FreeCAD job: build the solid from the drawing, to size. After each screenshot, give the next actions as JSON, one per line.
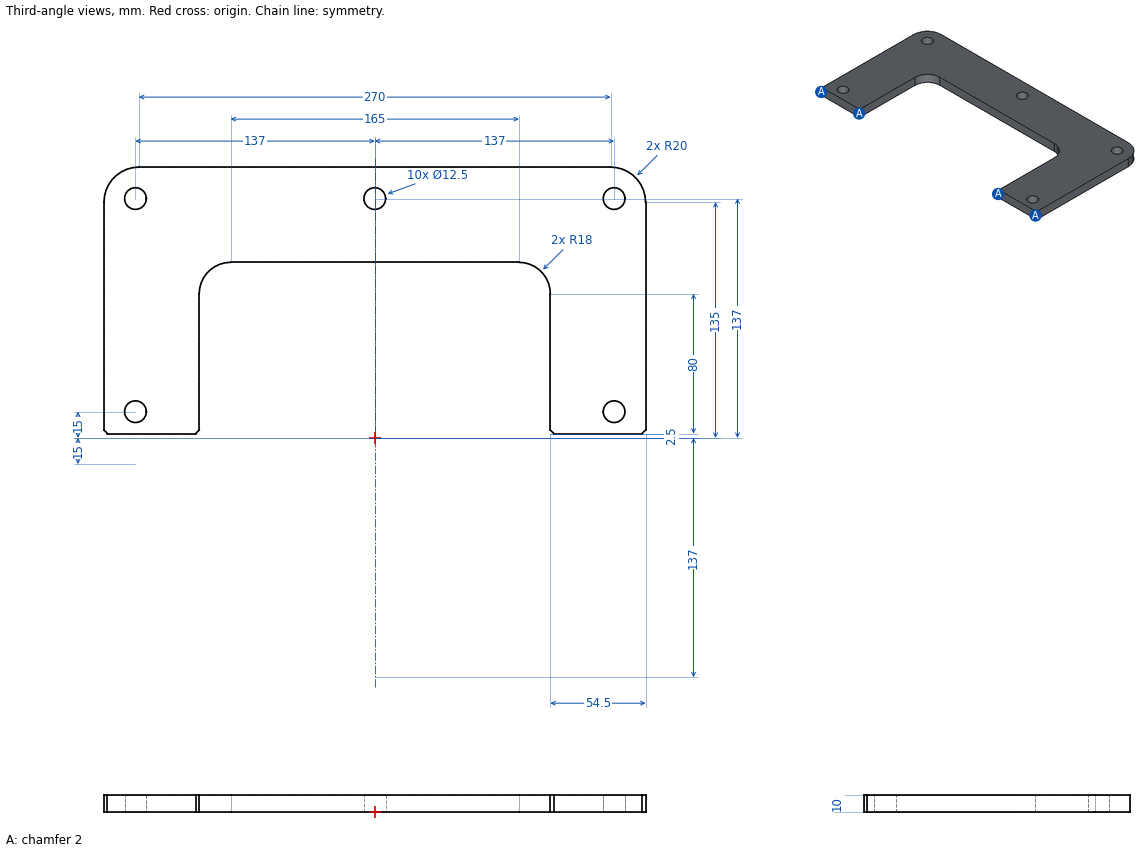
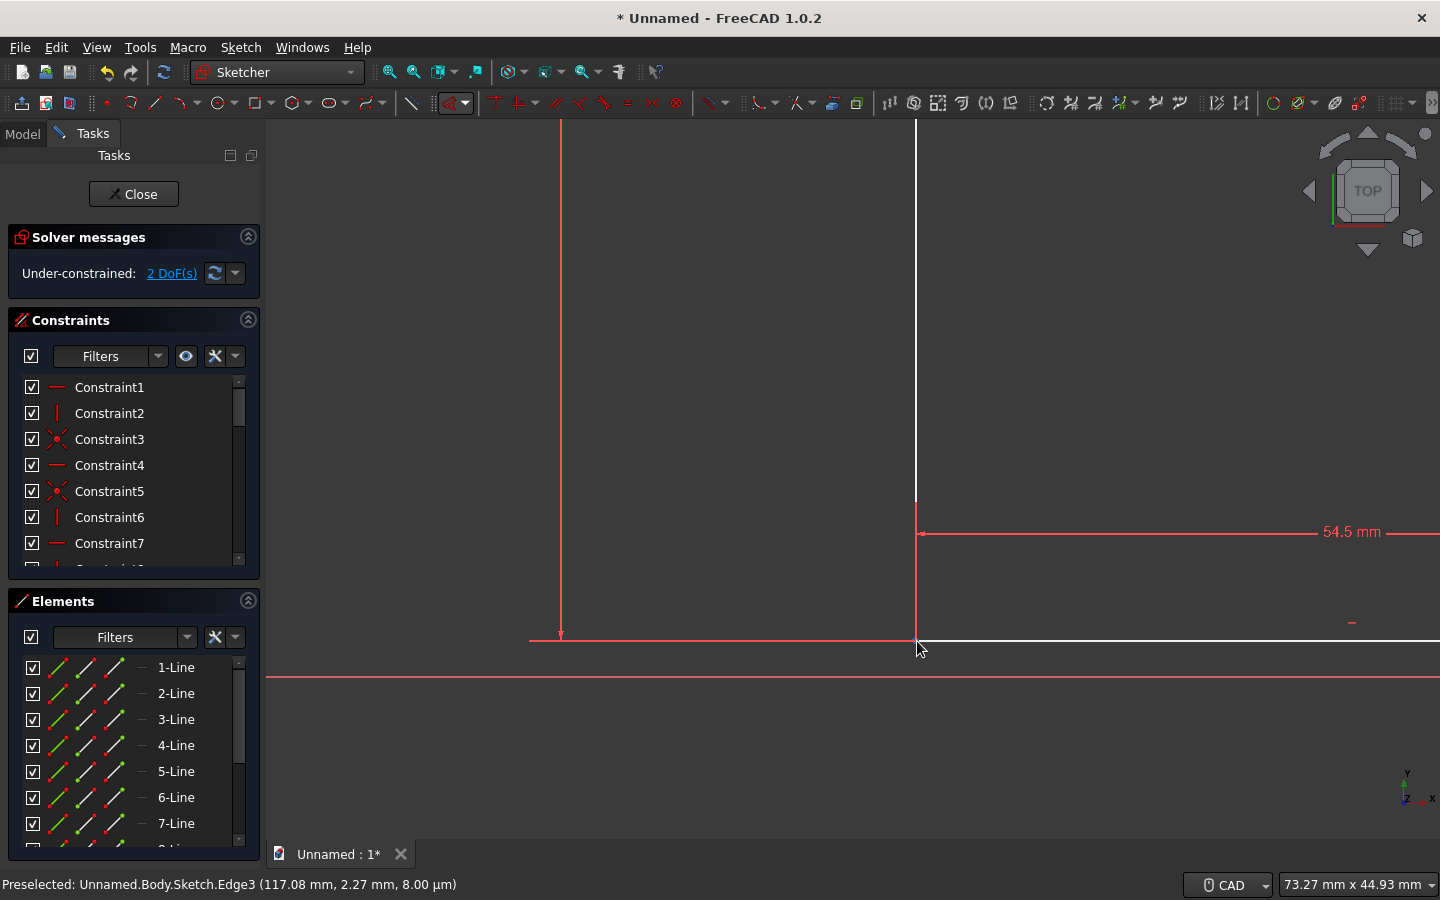
{"action": "left_click", "coordinate": [916, 641]}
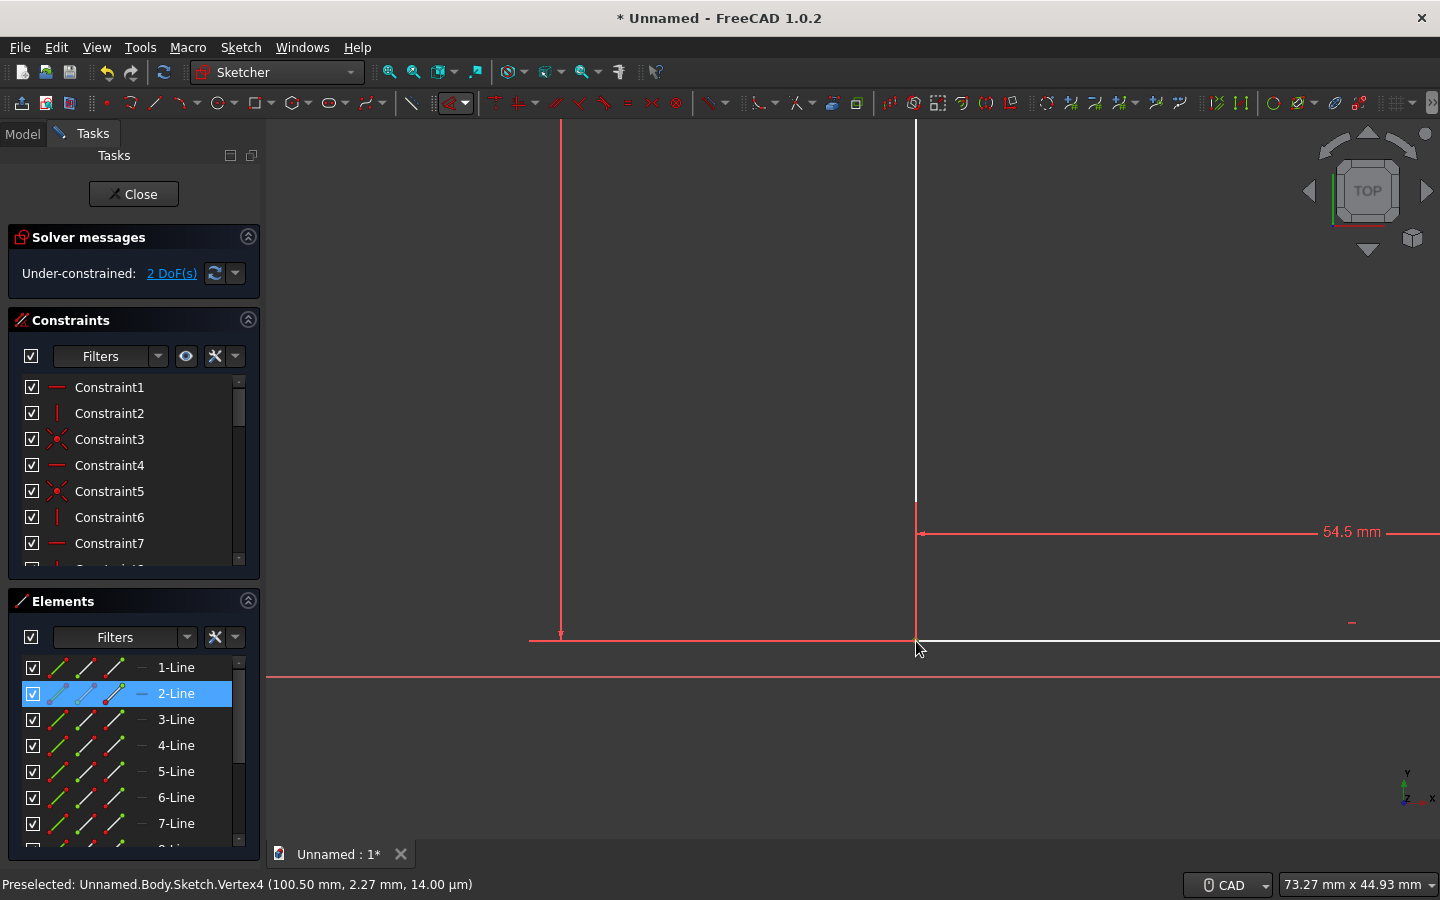
{"action": "key", "text": "i"}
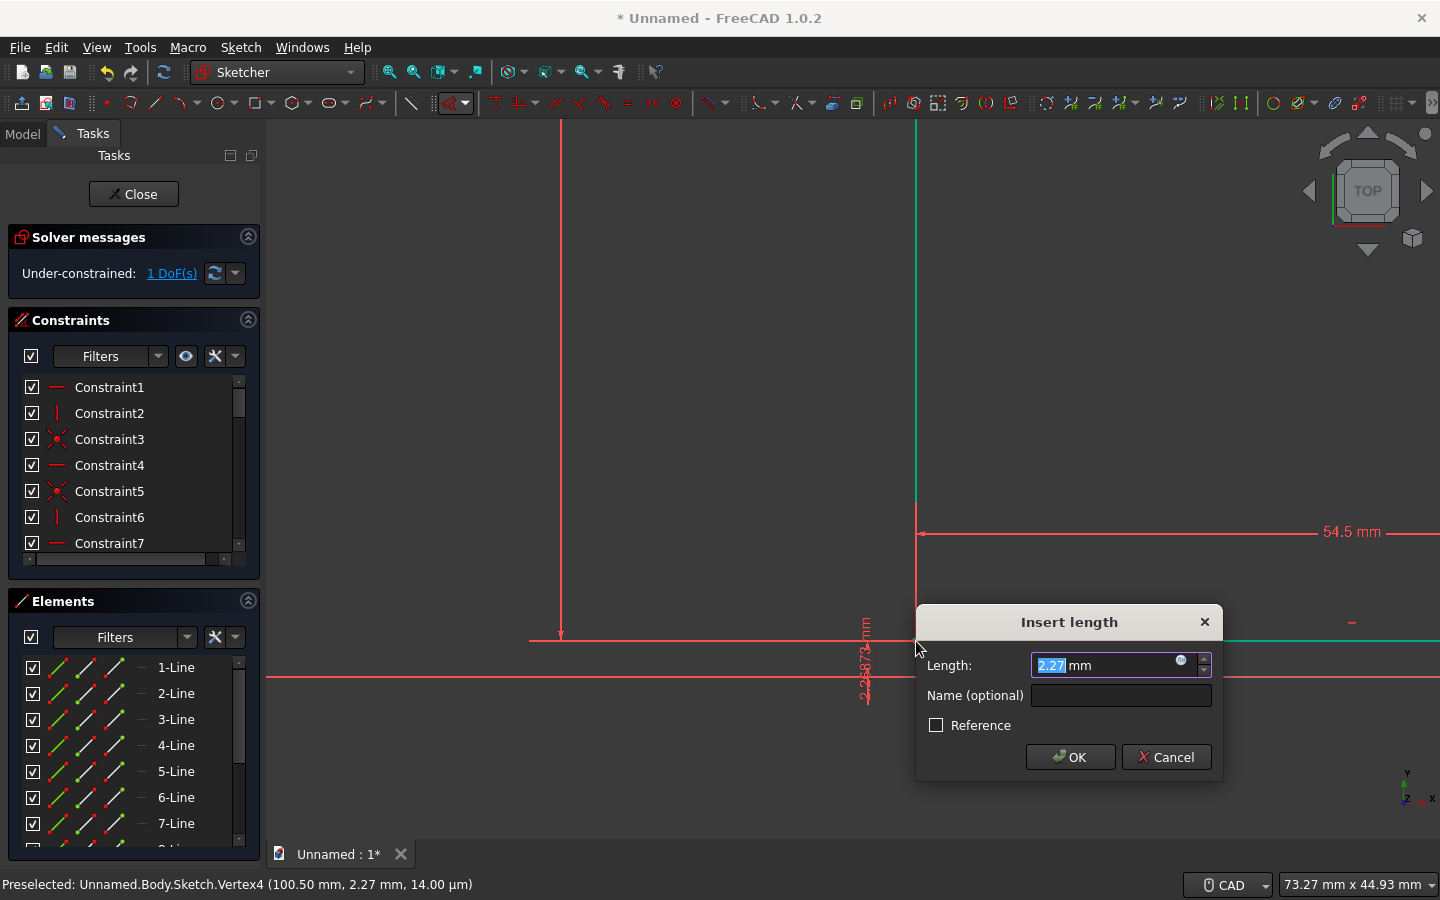
{"action": "type", "text": "2.5"}
{"action": "key", "text": "Return"}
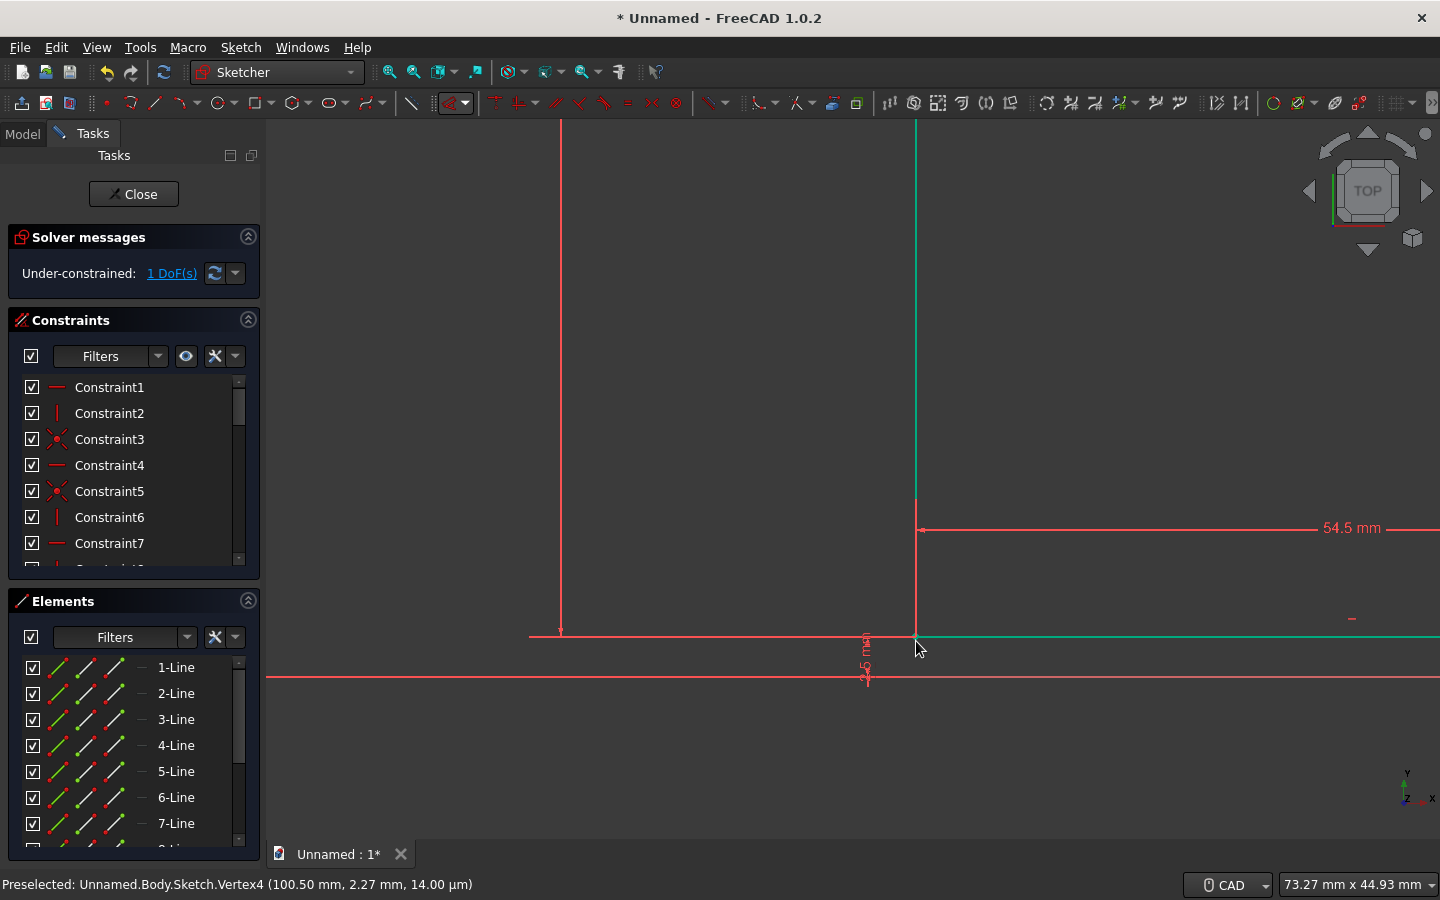
{"action": "scroll", "coordinate": [1016, 642], "scroll_direction": "down", "scroll_amount": 10}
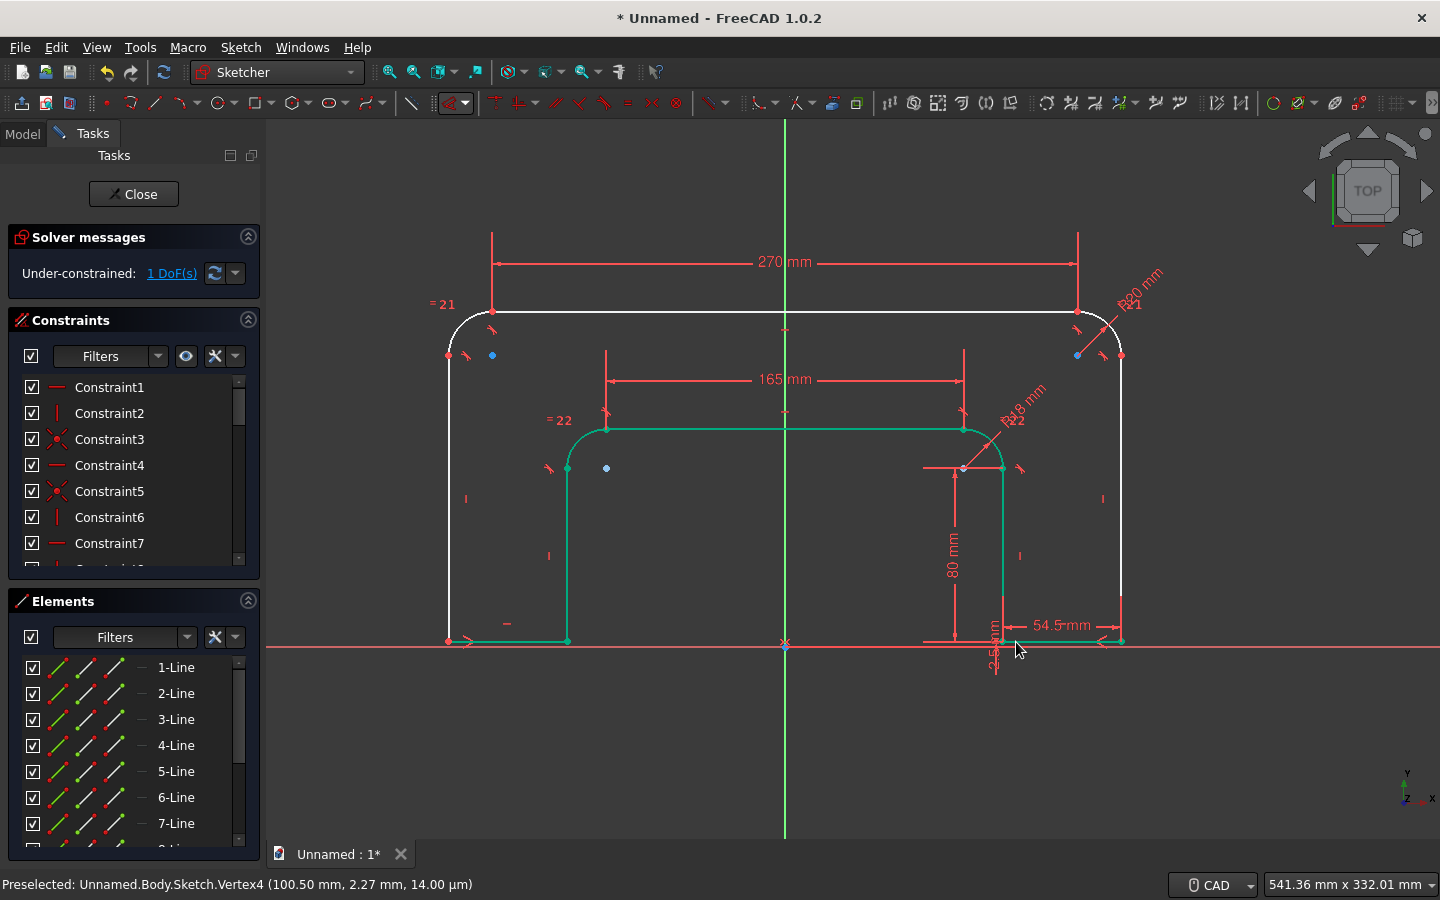
{"action": "left_click", "coordinate": [1121, 355]}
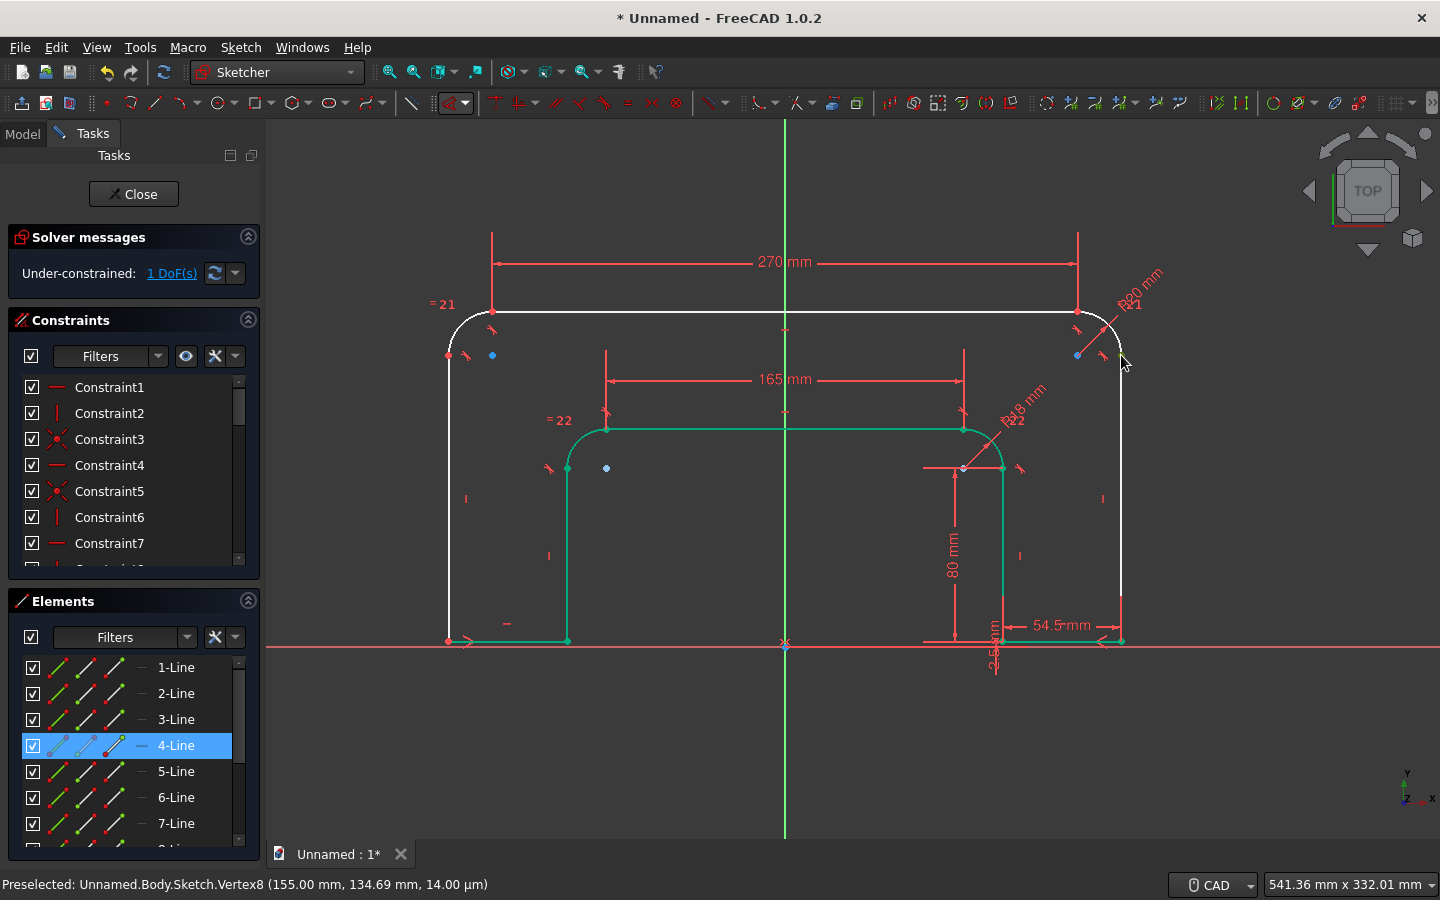
{"action": "key", "text": "i"}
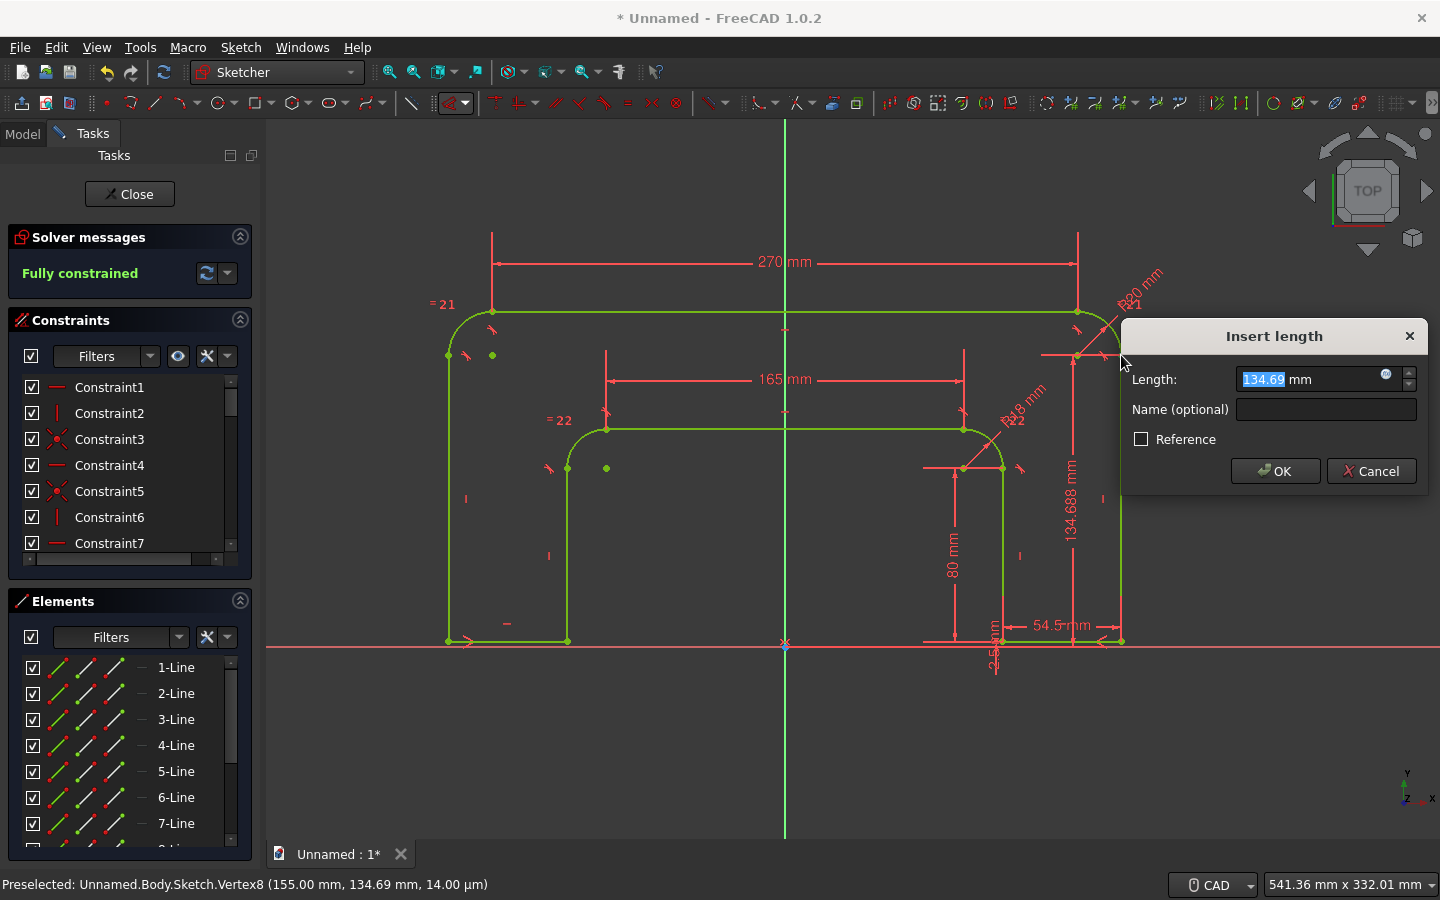
{"action": "type", "text": "135"}
{"action": "key", "text": "Return"}